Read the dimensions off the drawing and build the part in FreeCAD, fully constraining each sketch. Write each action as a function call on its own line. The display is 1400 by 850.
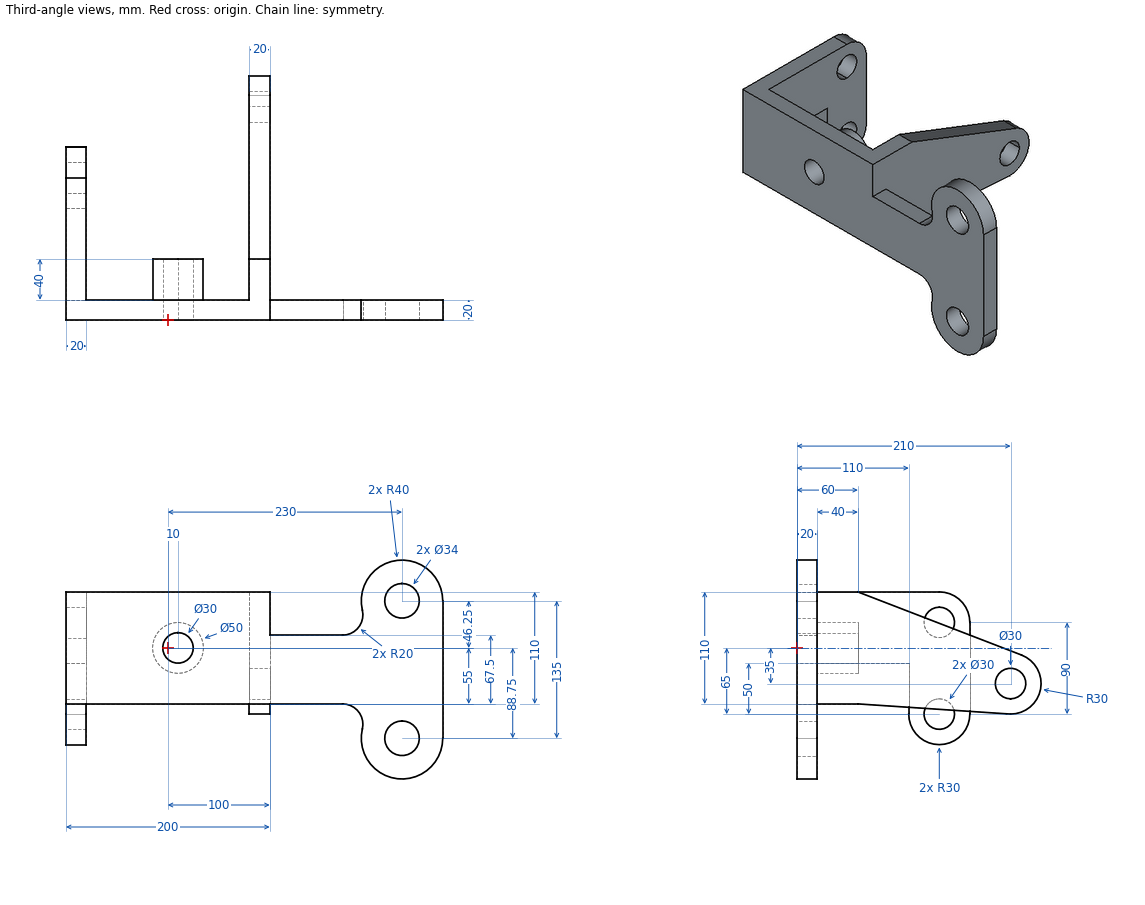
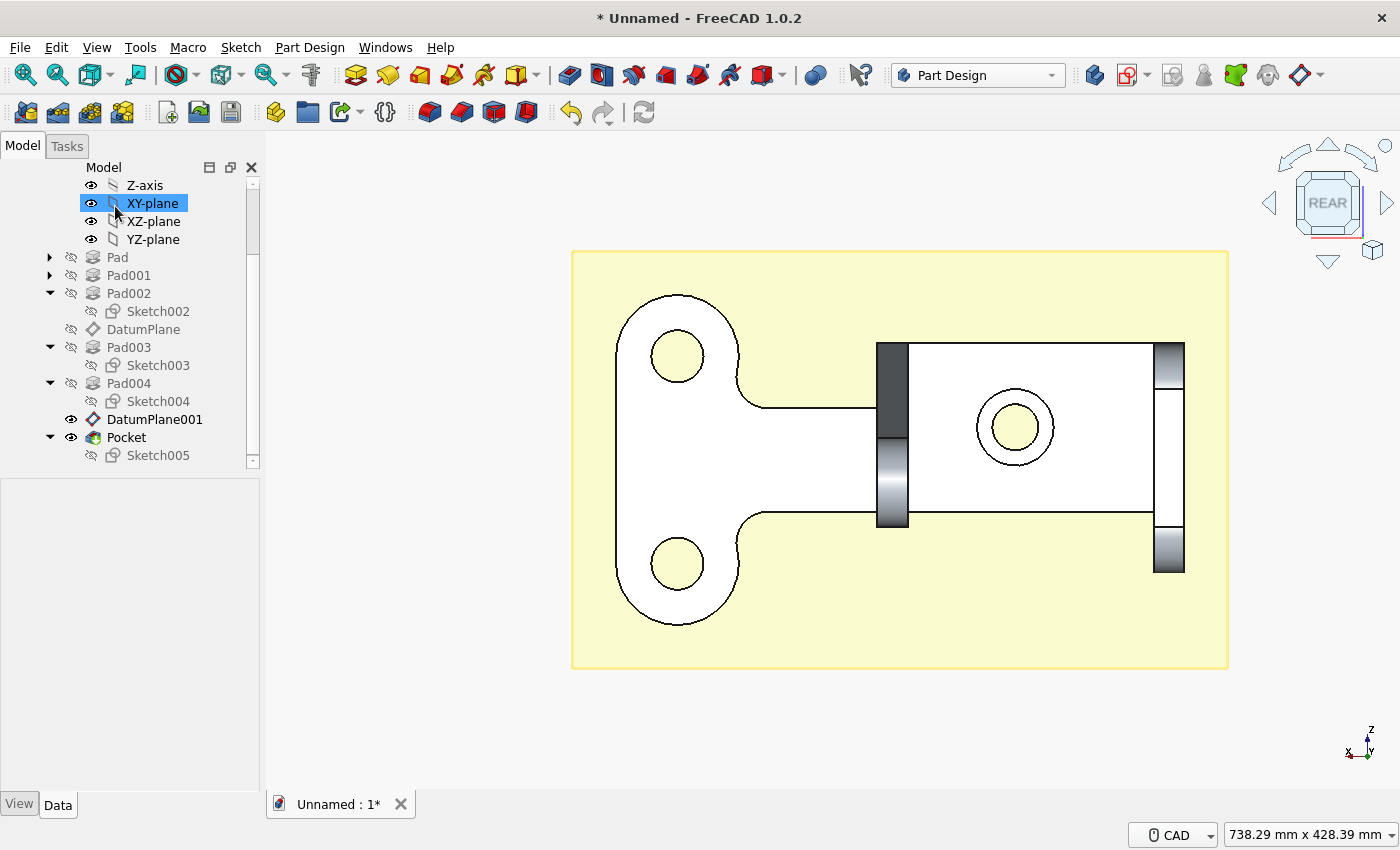
click(116, 419)
key(space)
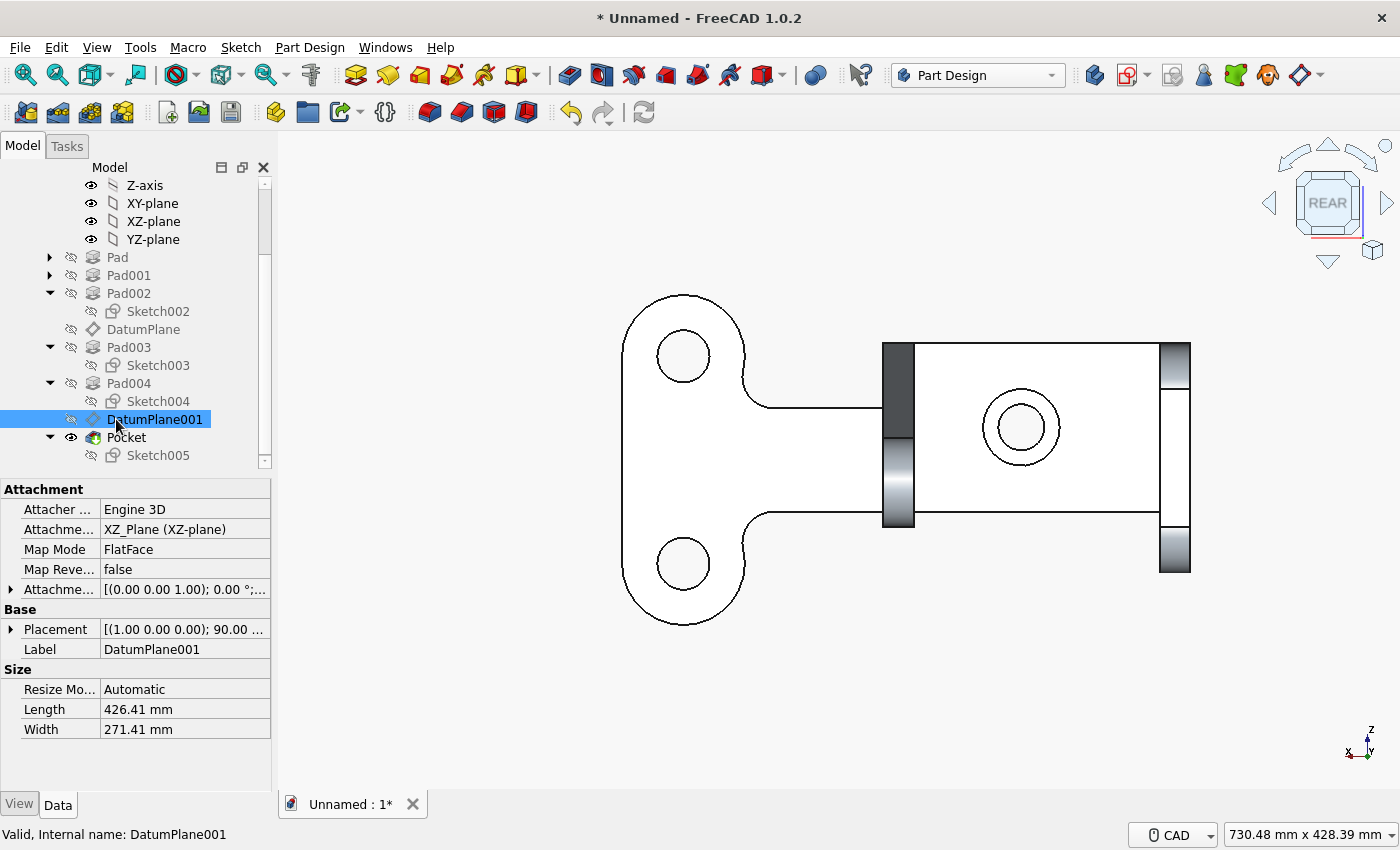
key(0)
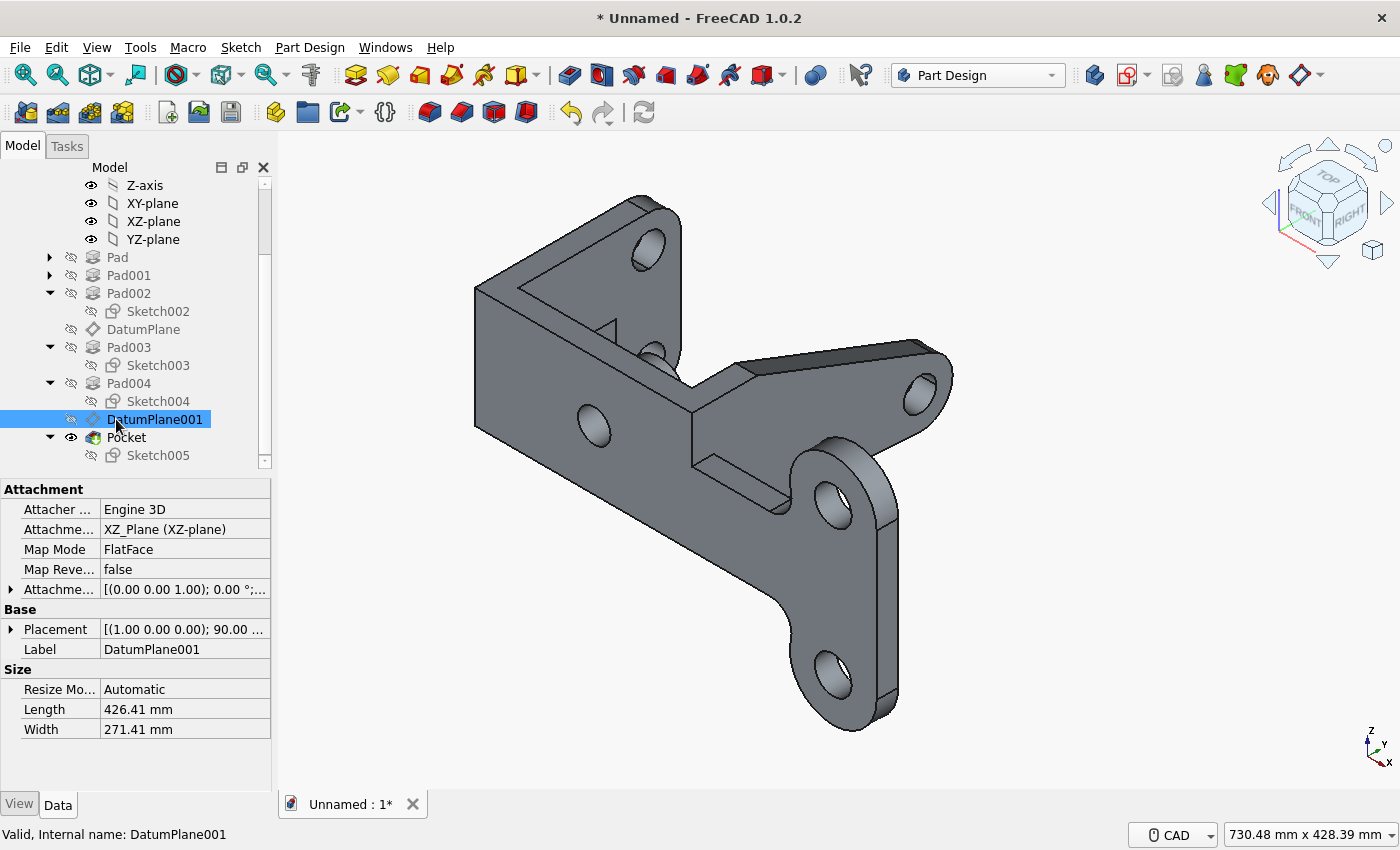
key(v)
key(f)